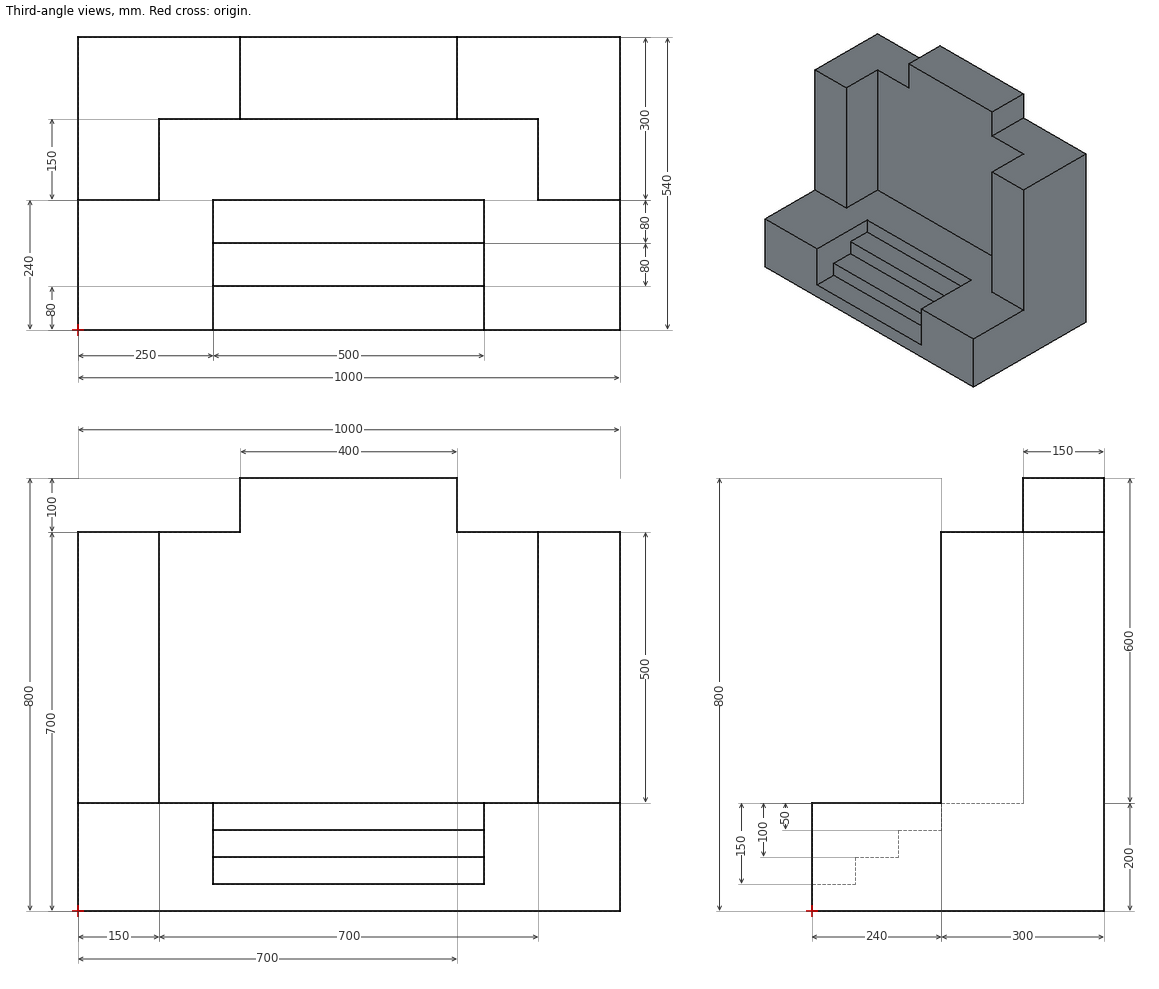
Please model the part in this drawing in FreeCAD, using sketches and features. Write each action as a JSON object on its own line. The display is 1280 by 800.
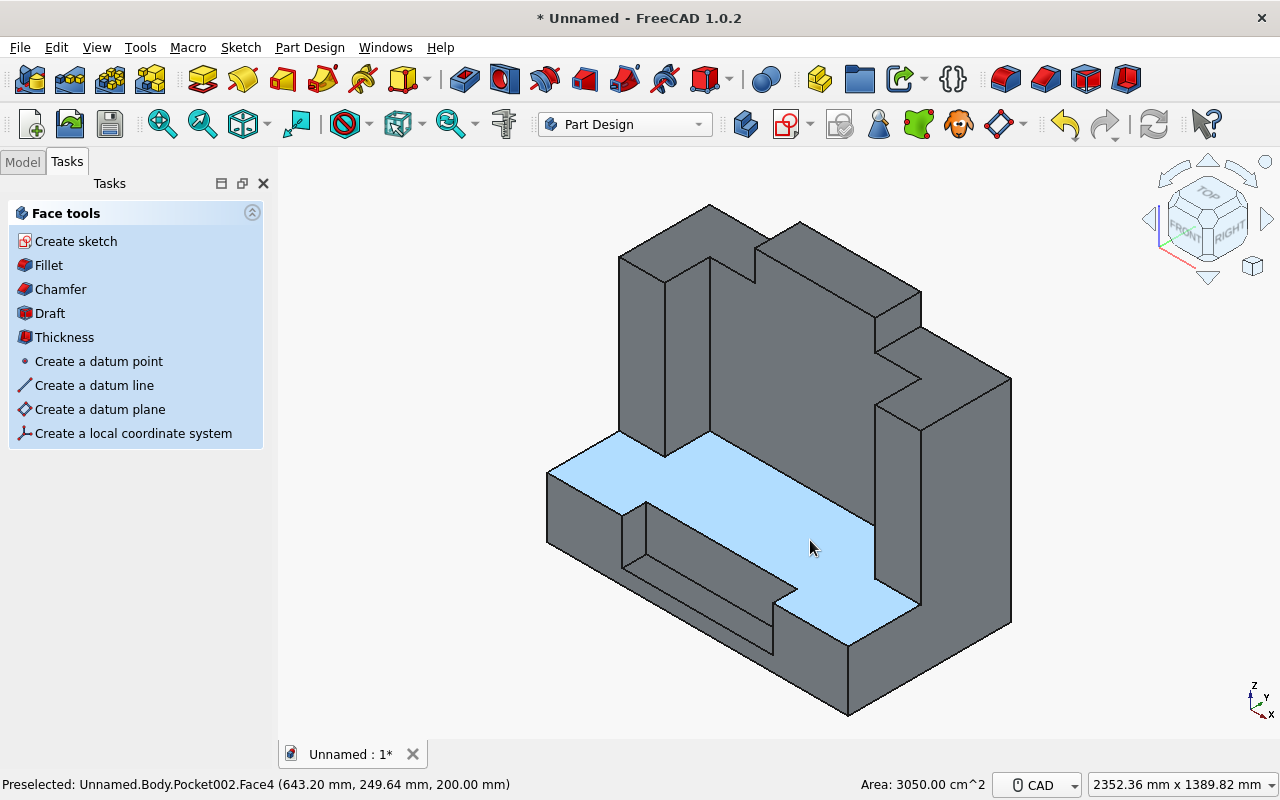
{"action": "left_click", "coordinate": [786, 124]}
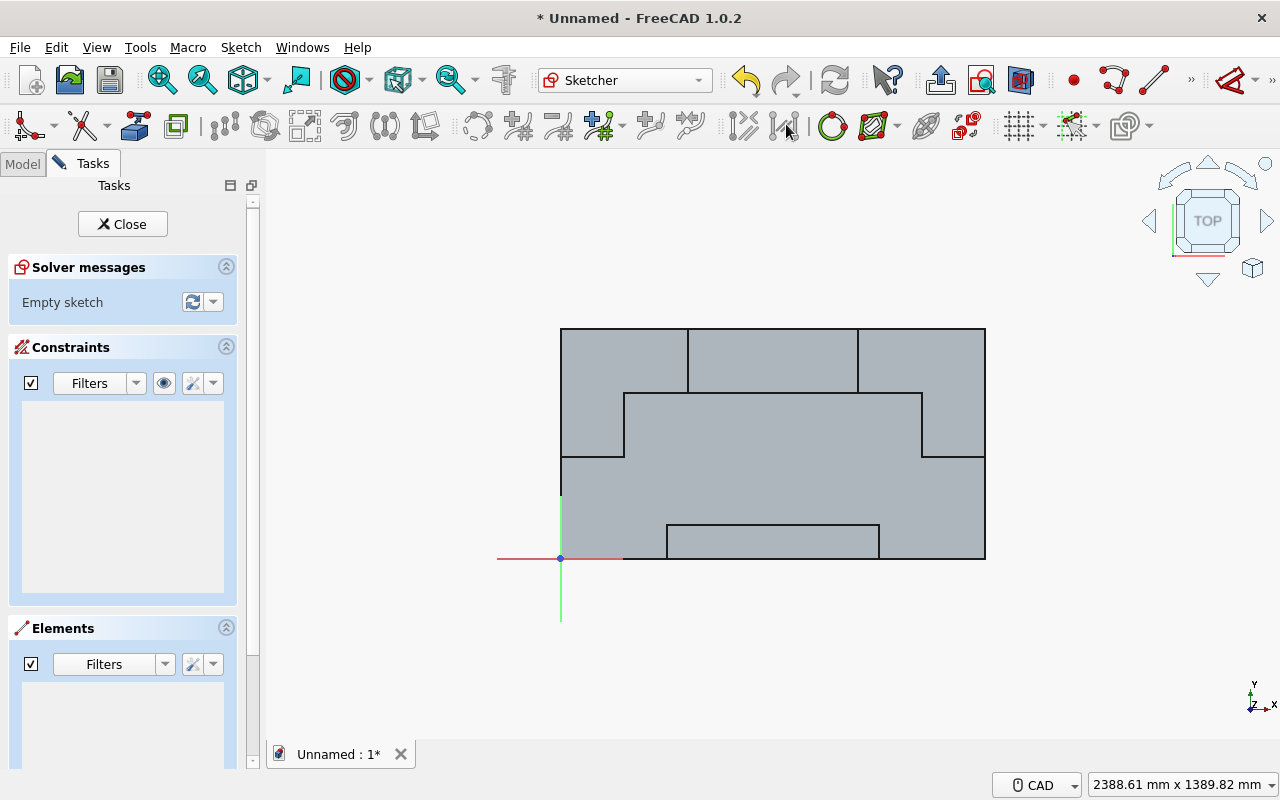
{"action": "left_click", "coordinate": [1022, 80]}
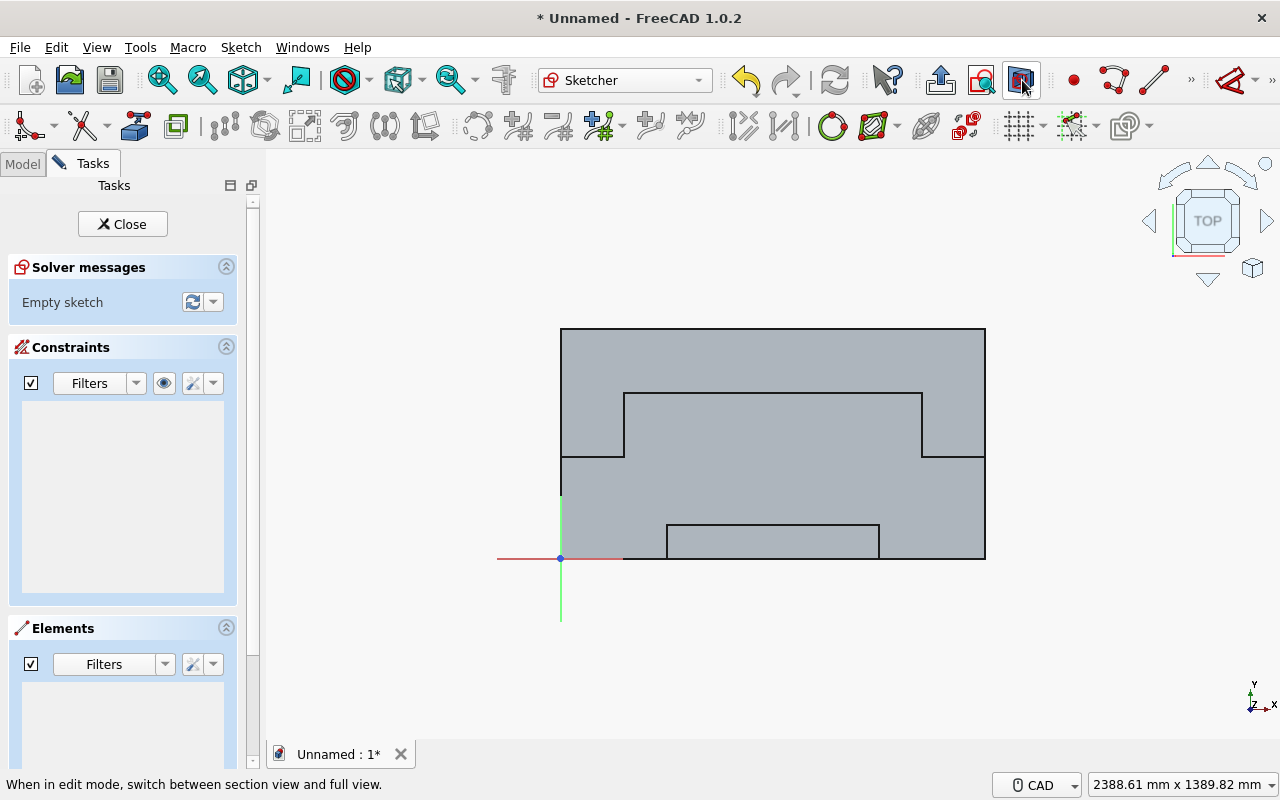
{"action": "scroll", "coordinate": [739, 623], "scroll_direction": "up", "scroll_amount": 3}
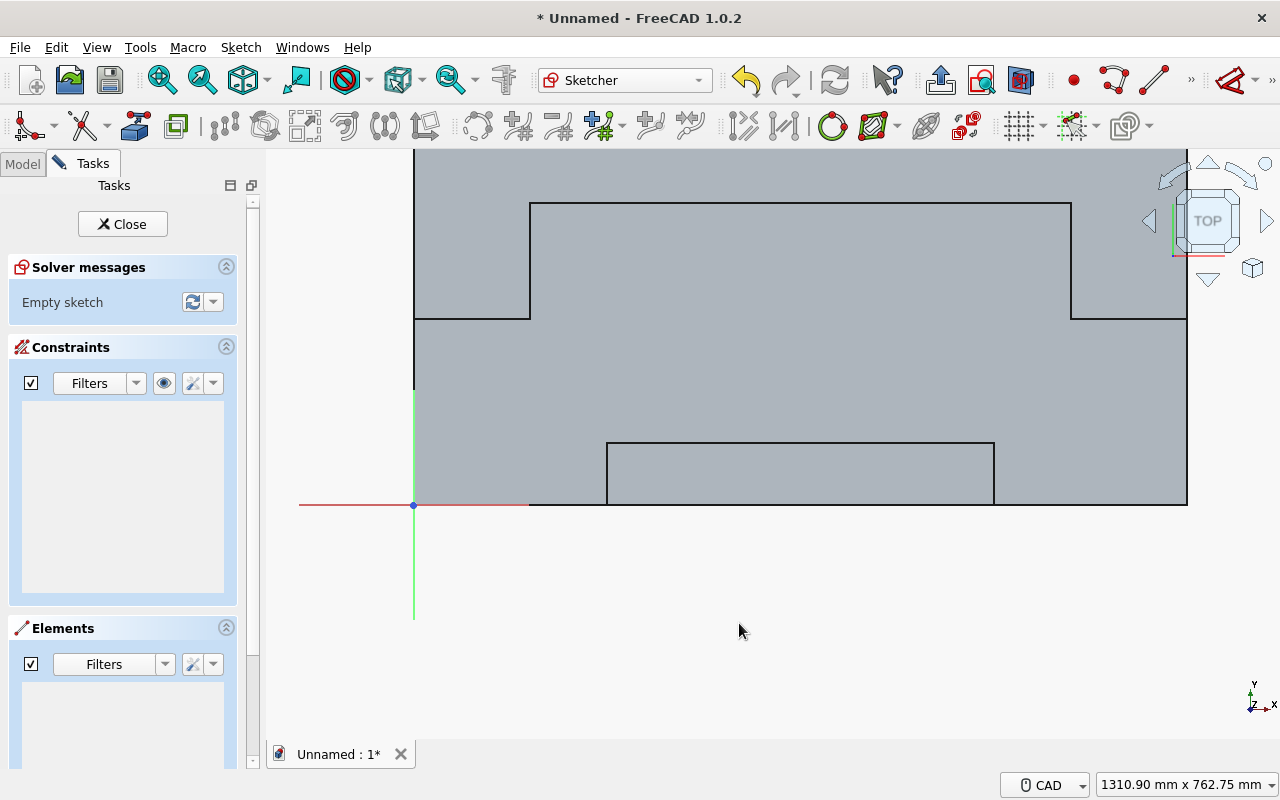
{"action": "key", "text": "g r"}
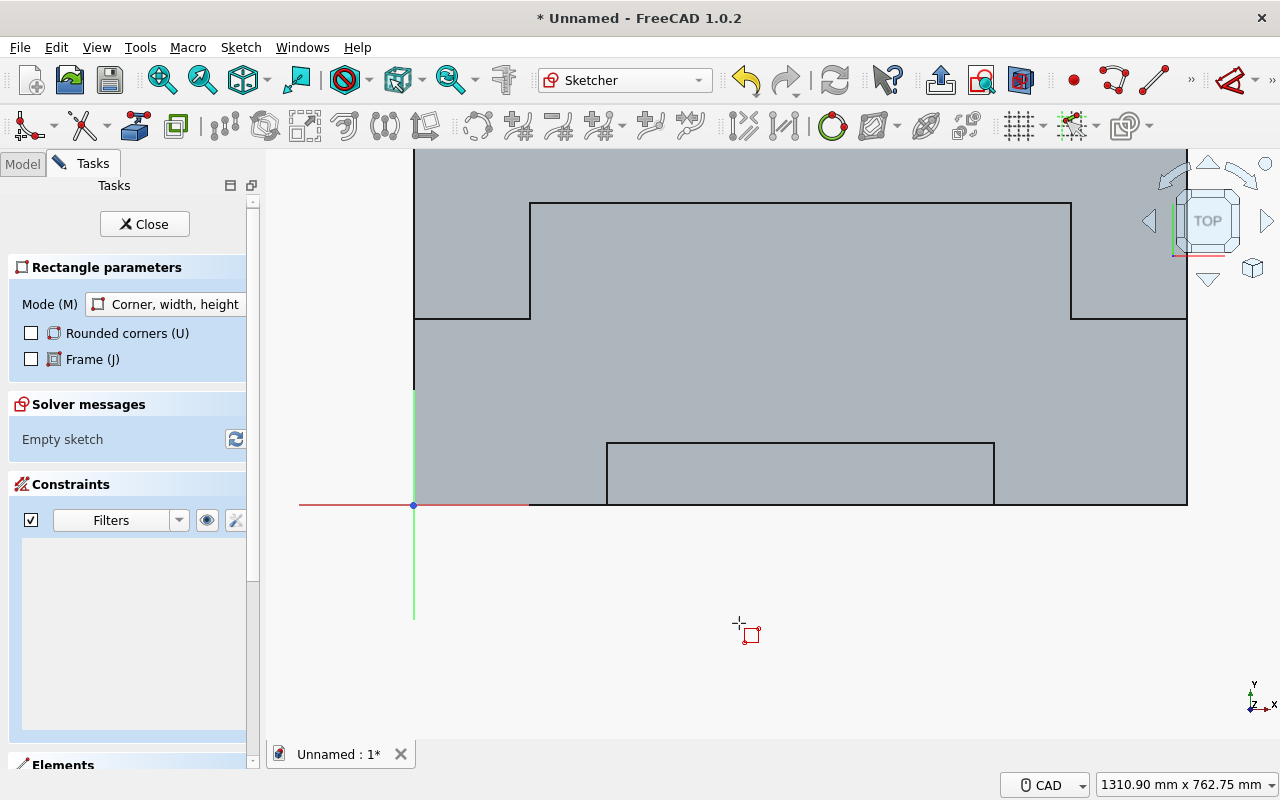
{"action": "left_click", "coordinate": [607, 381]}
{"action": "mouse_move", "coordinate": [994, 443]}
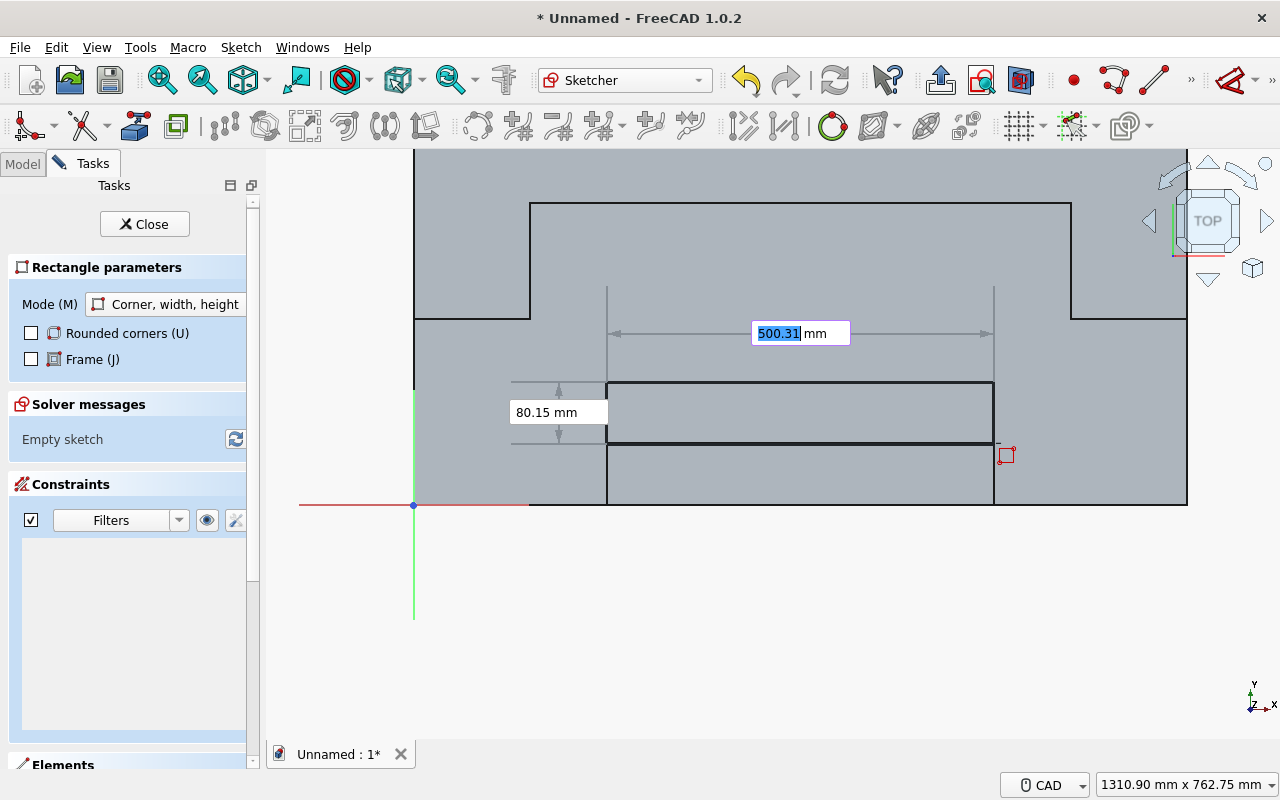
{"action": "type", "text": "500"}
{"action": "key", "text": "Tab"}
{"action": "type", "text": "80"}
{"action": "key", "text": "Return"}
{"action": "key", "text": "Escape"}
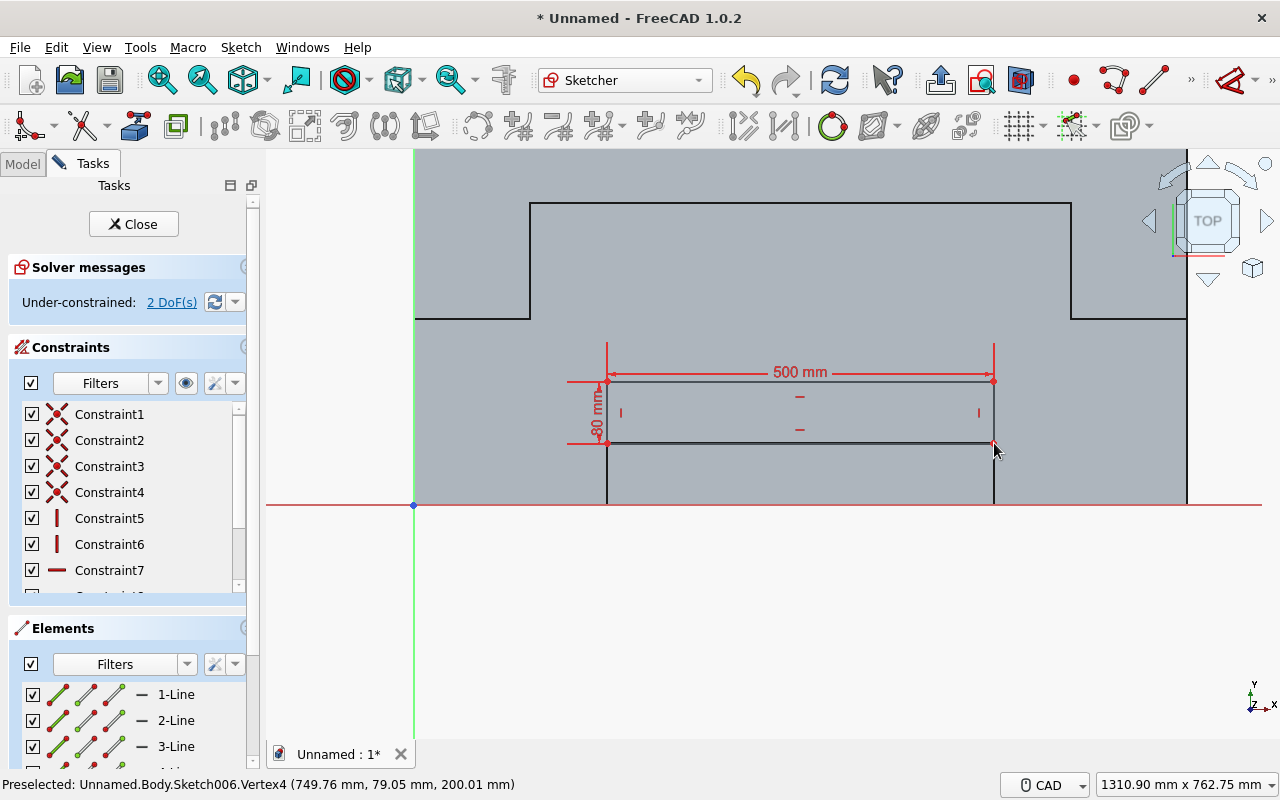
{"action": "left_click", "coordinate": [1230, 80]}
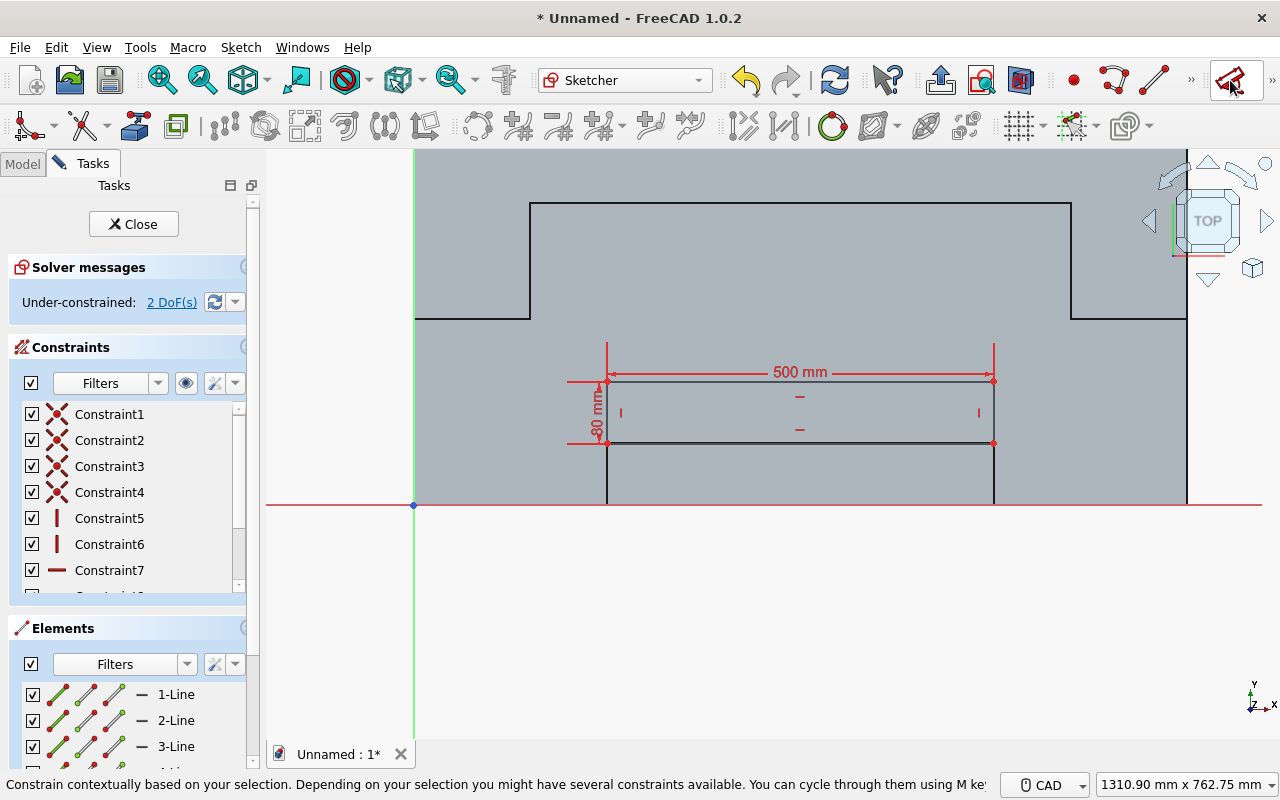
{"action": "left_click", "coordinate": [607, 444]}
{"action": "left_click", "coordinate": [380, 474]}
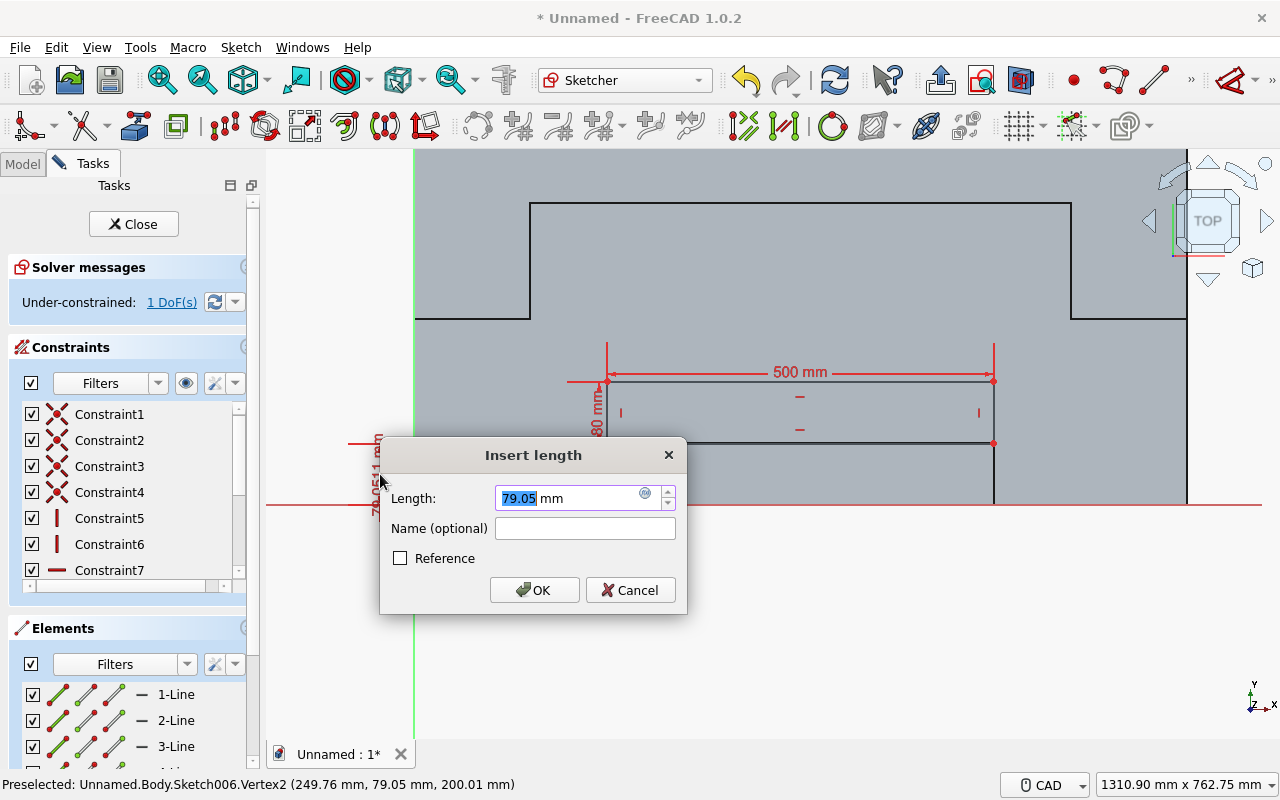
{"action": "type", "text": "80"}
{"action": "key", "text": "Return"}